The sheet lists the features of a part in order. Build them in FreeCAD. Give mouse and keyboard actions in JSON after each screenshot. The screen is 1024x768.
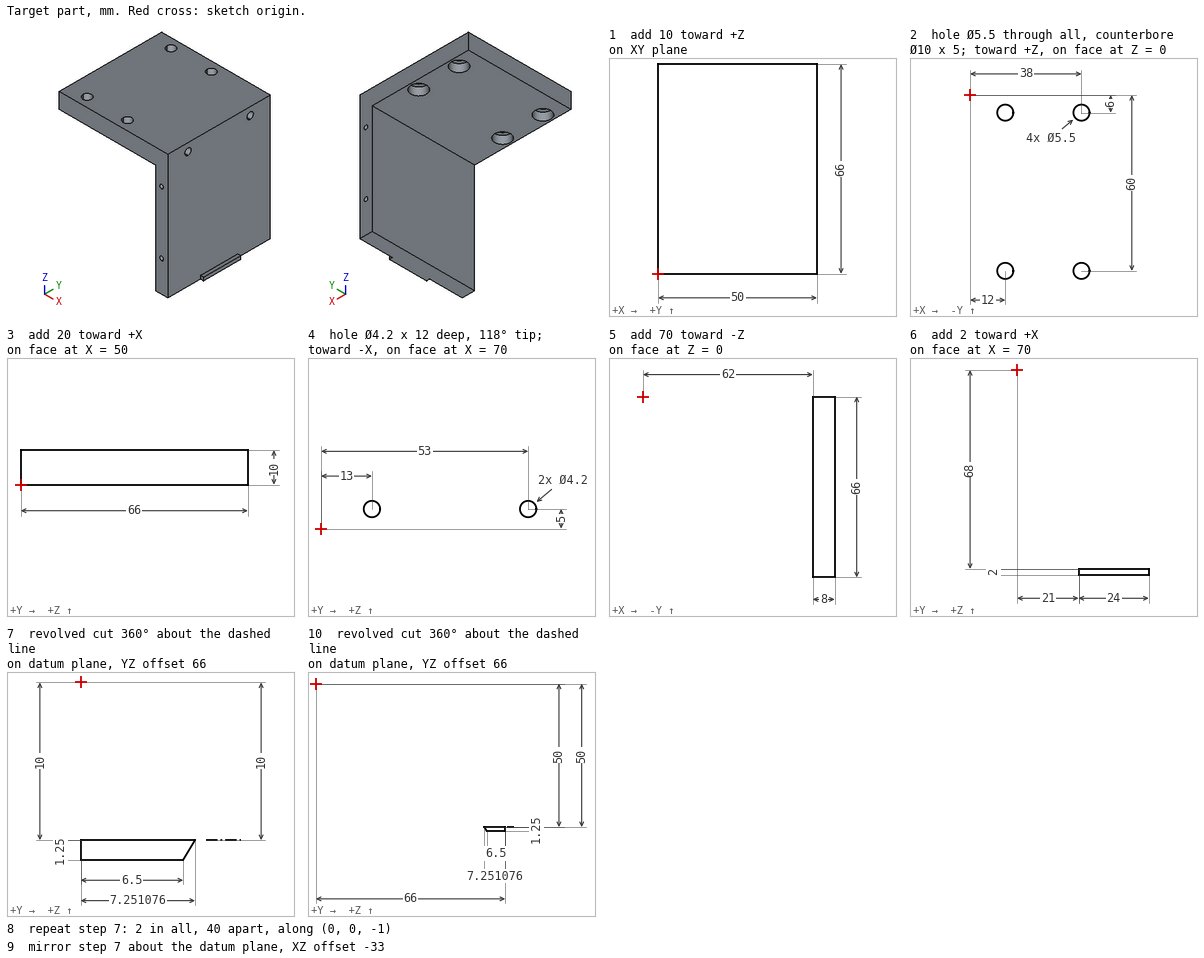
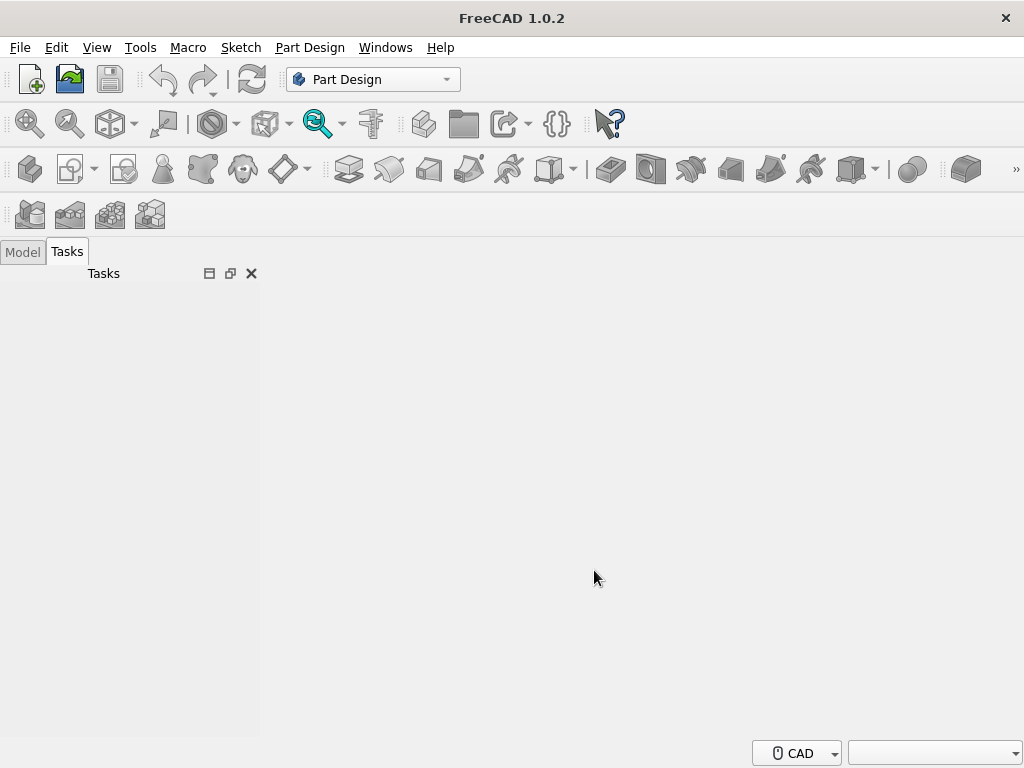
{"action": "key", "text": "ctrl+n"}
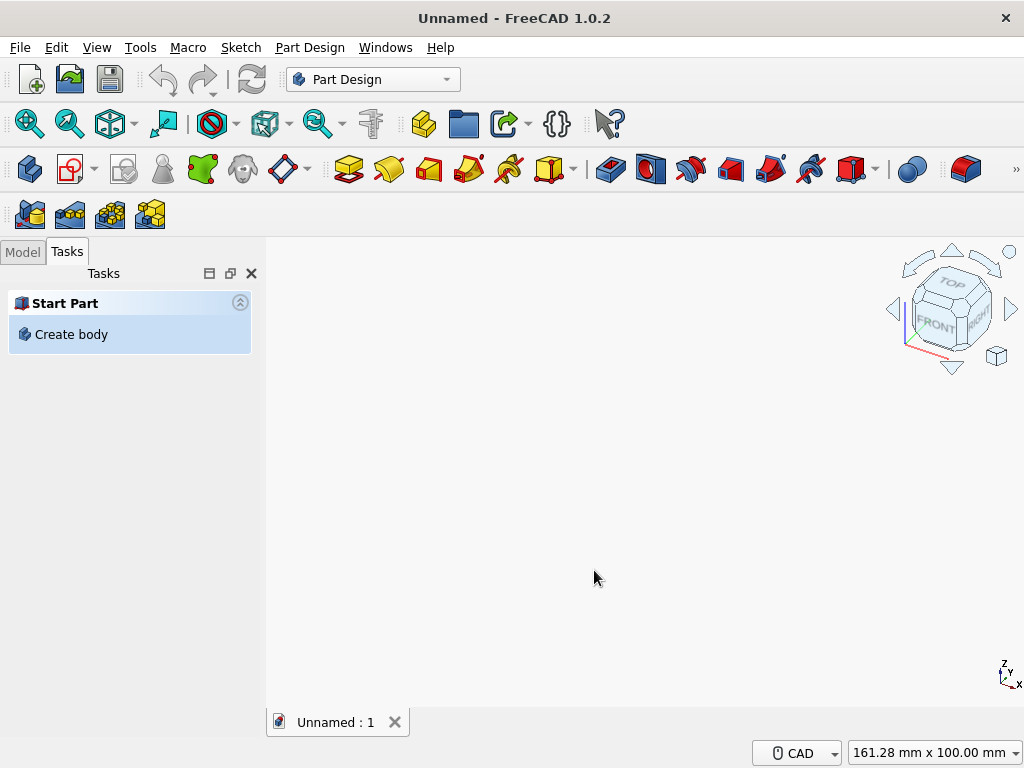
{"action": "left_click", "coordinate": [70, 170]}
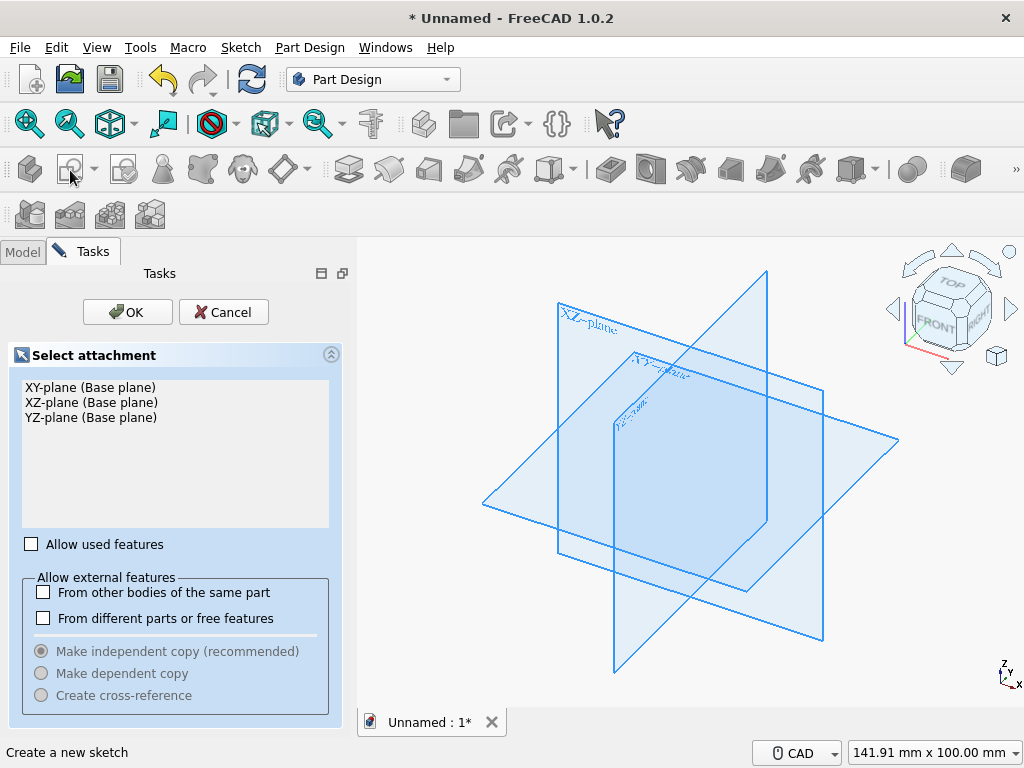
{"action": "left_click", "coordinate": [82, 388]}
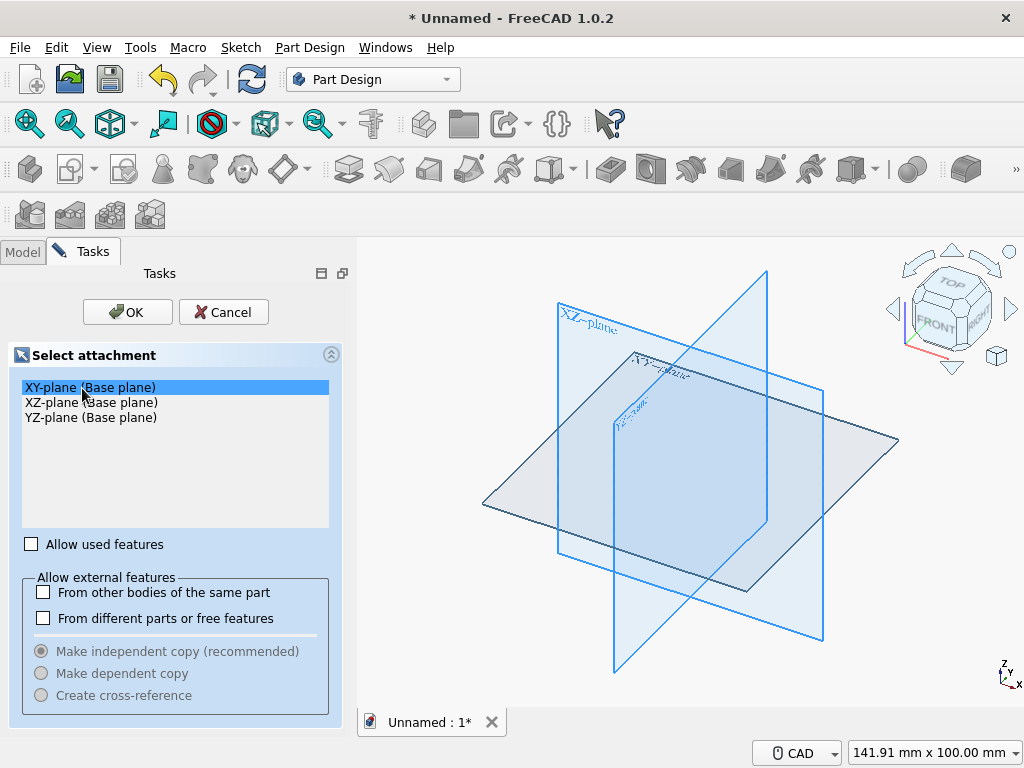
{"action": "left_click", "coordinate": [128, 312]}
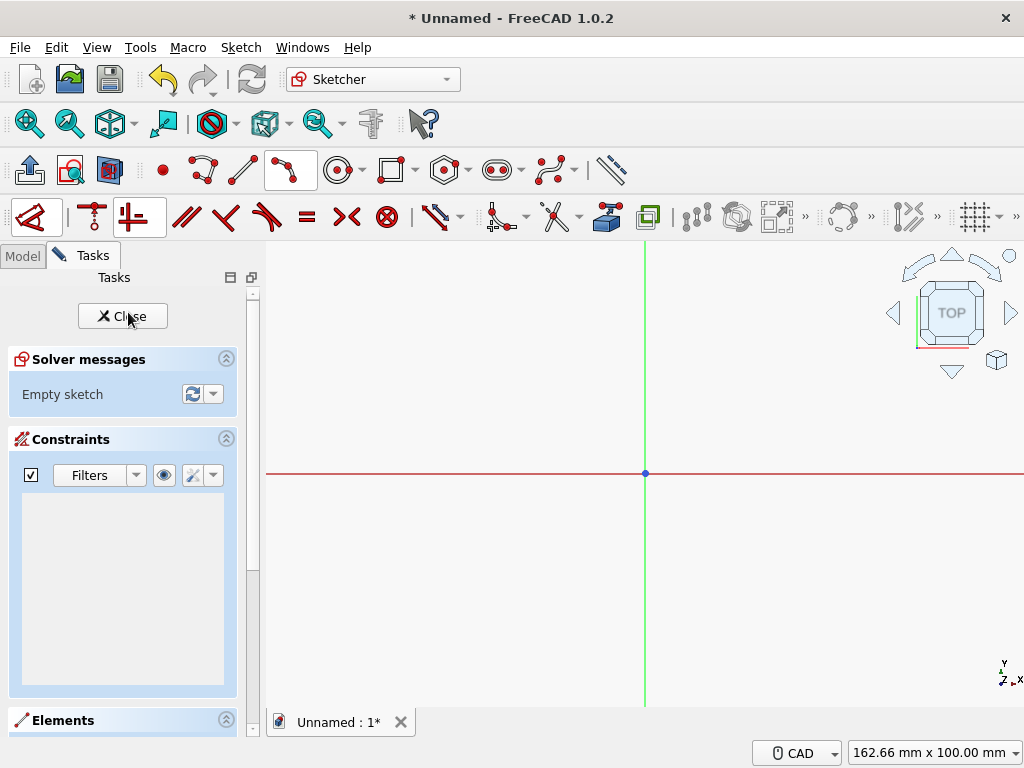
{"action": "scroll", "coordinate": [294, 679], "scroll_direction": "down", "scroll_amount": 2}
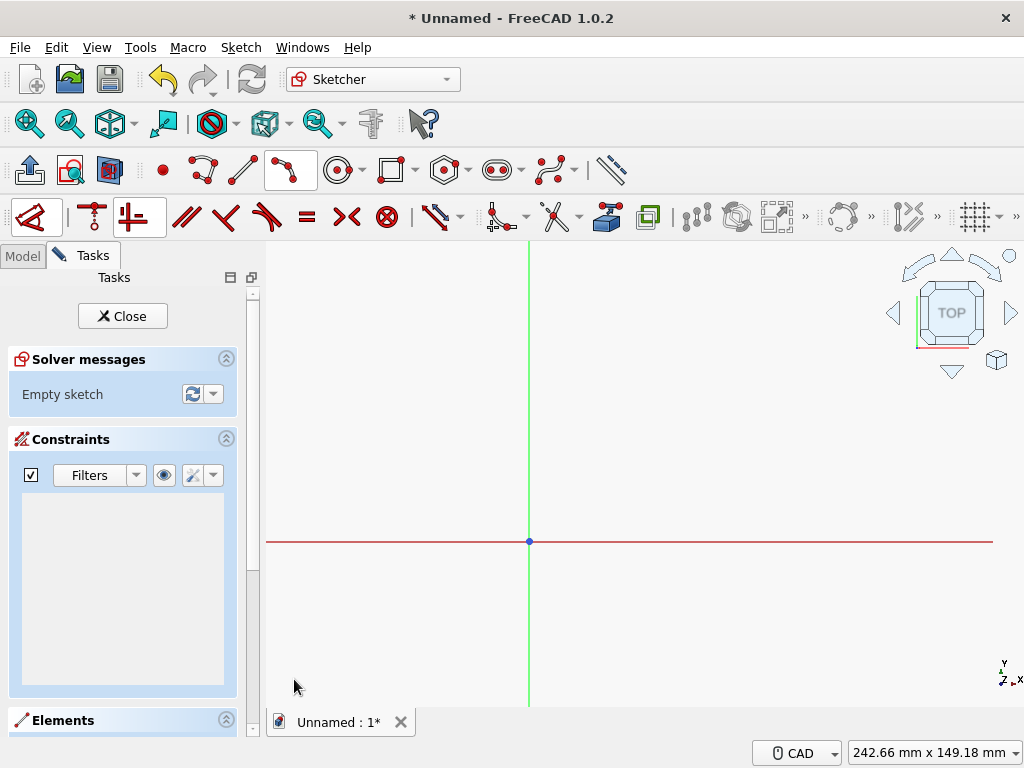
{"action": "scroll", "coordinate": [670, 367], "scroll_direction": "up", "scroll_amount": 2}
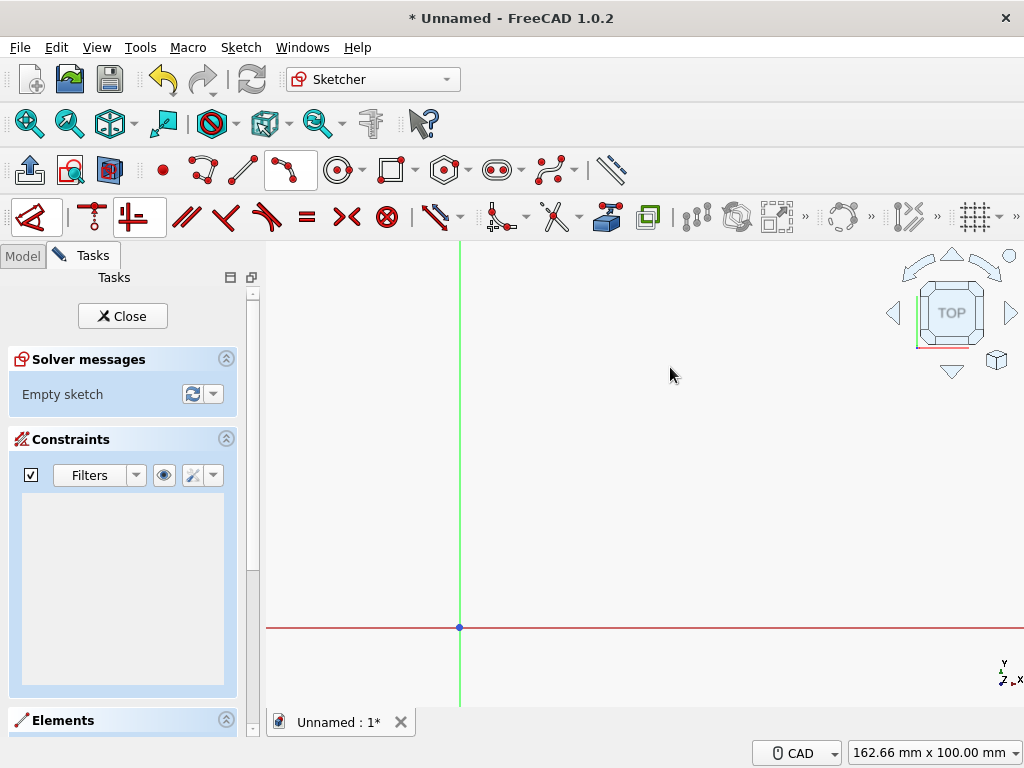
{"action": "key", "text": "g r"}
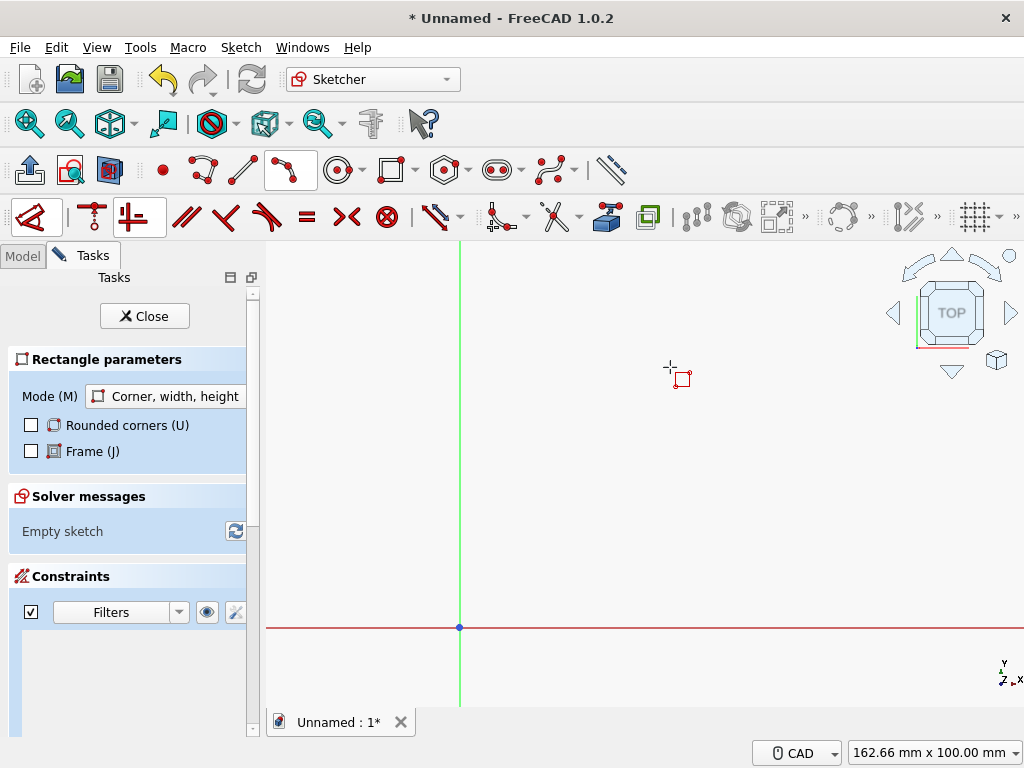
{"action": "left_click", "coordinate": [460, 628]}
{"action": "left_click", "coordinate": [693, 320]}
{"action": "key", "text": "Escape"}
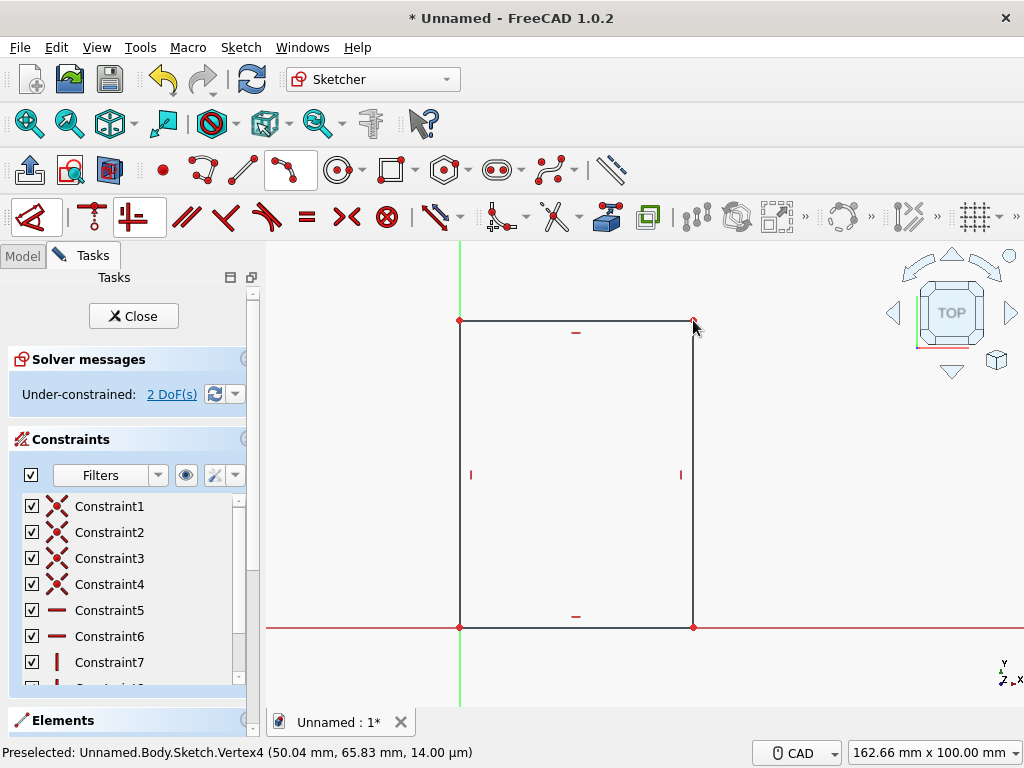
{"action": "left_click", "coordinate": [530, 628]}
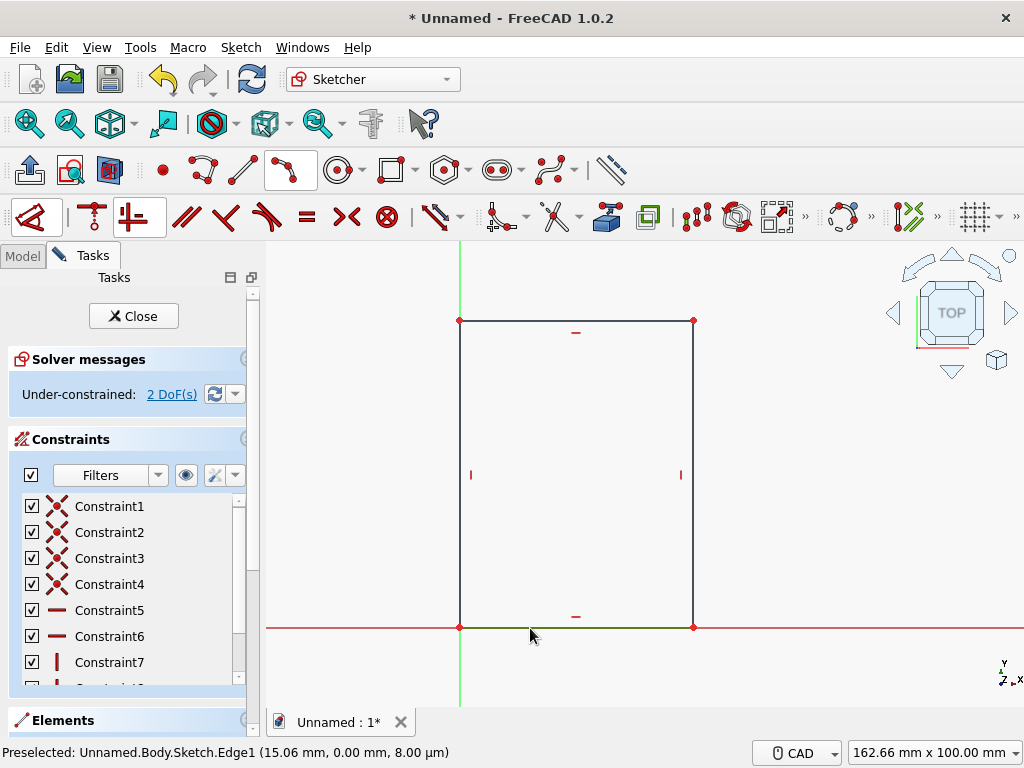
{"action": "key", "text": "l"}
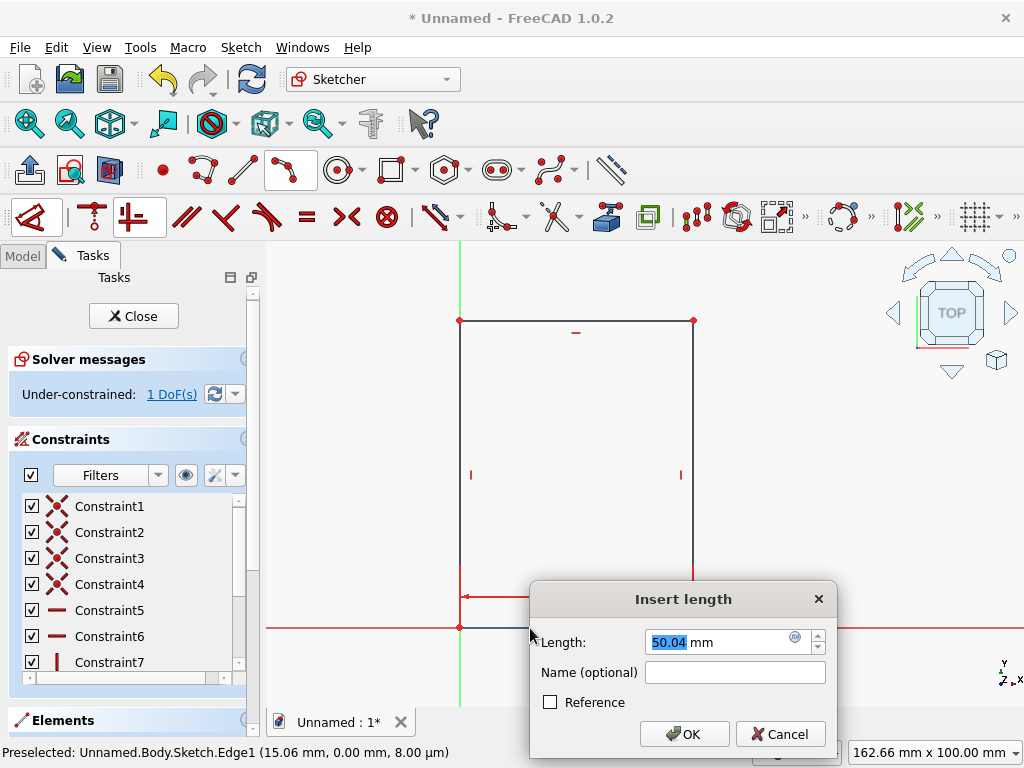
{"action": "type", "text": "50"}
{"action": "key", "text": "Return"}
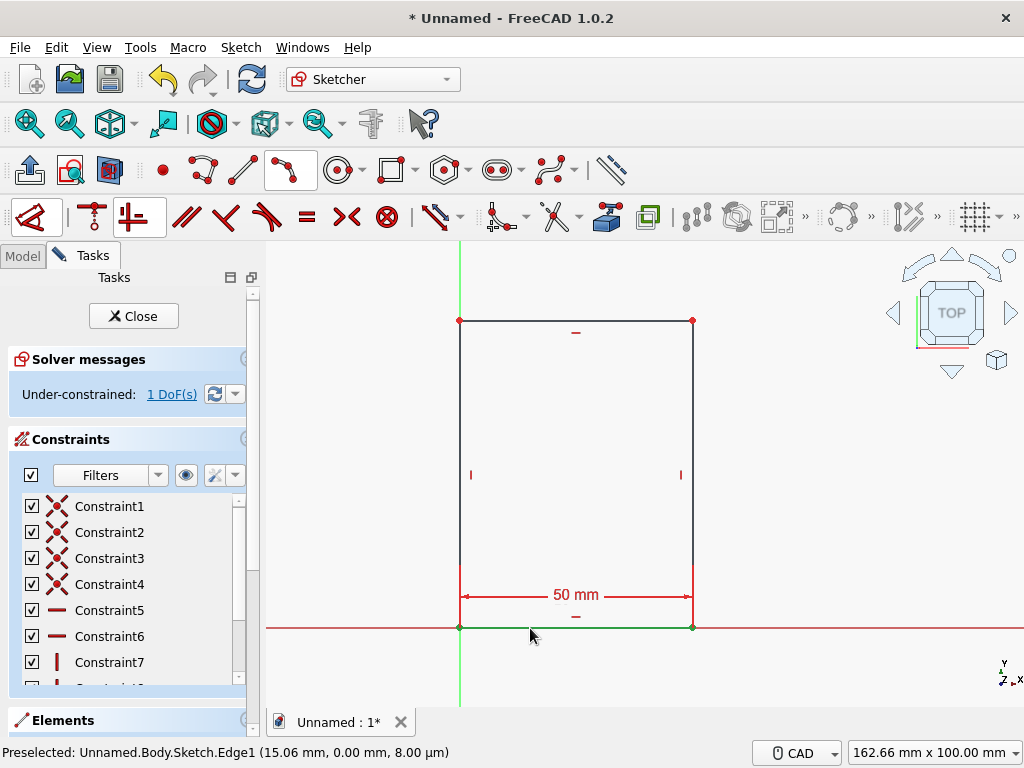
{"action": "left_click", "coordinate": [693, 536]}